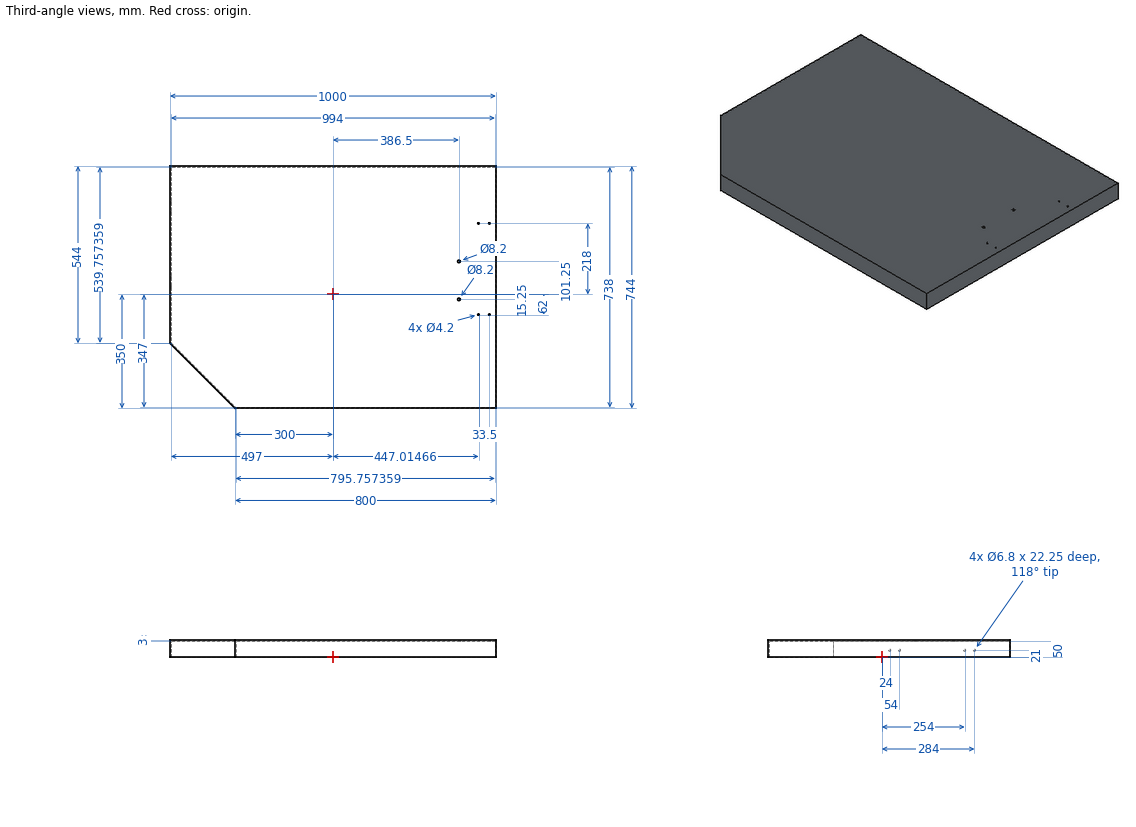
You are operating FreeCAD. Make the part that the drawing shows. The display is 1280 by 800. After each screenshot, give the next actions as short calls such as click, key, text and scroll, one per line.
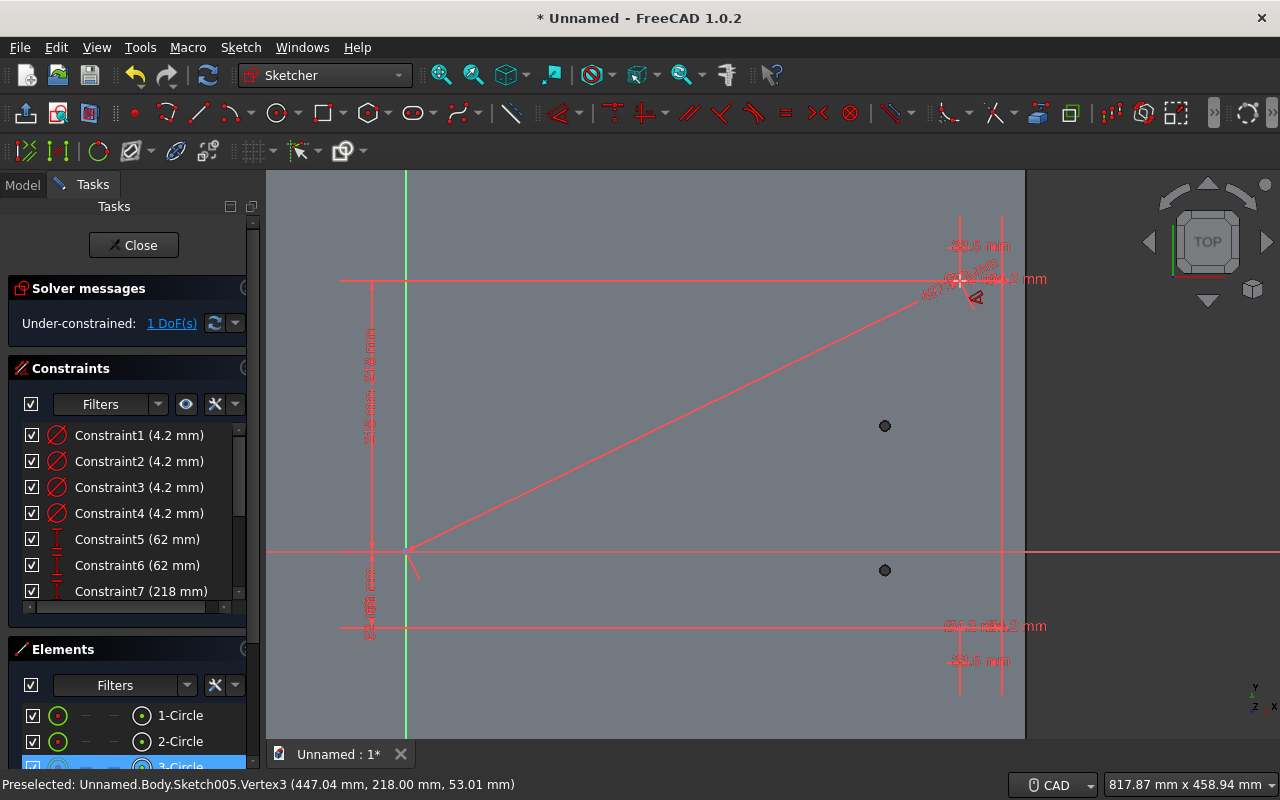
click(1002, 281)
click(981, 315)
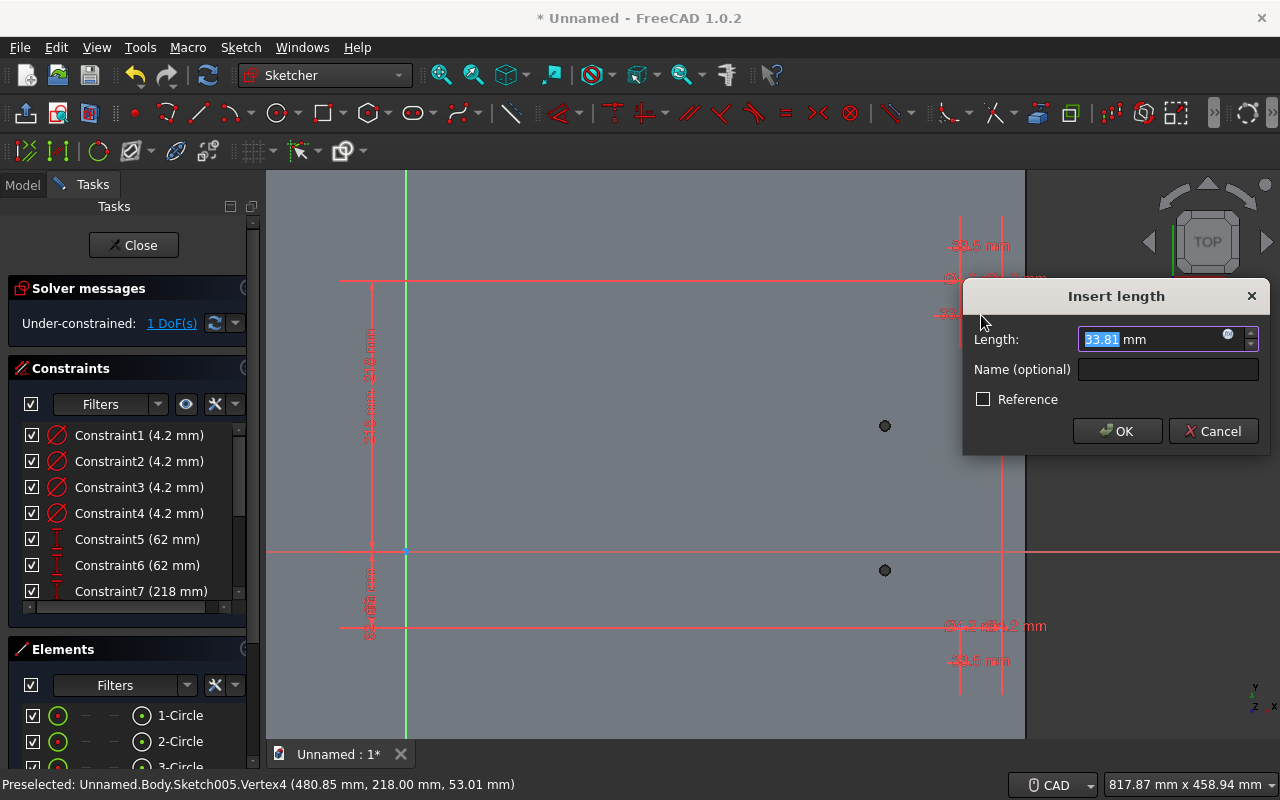
text(33.5)
key(Return)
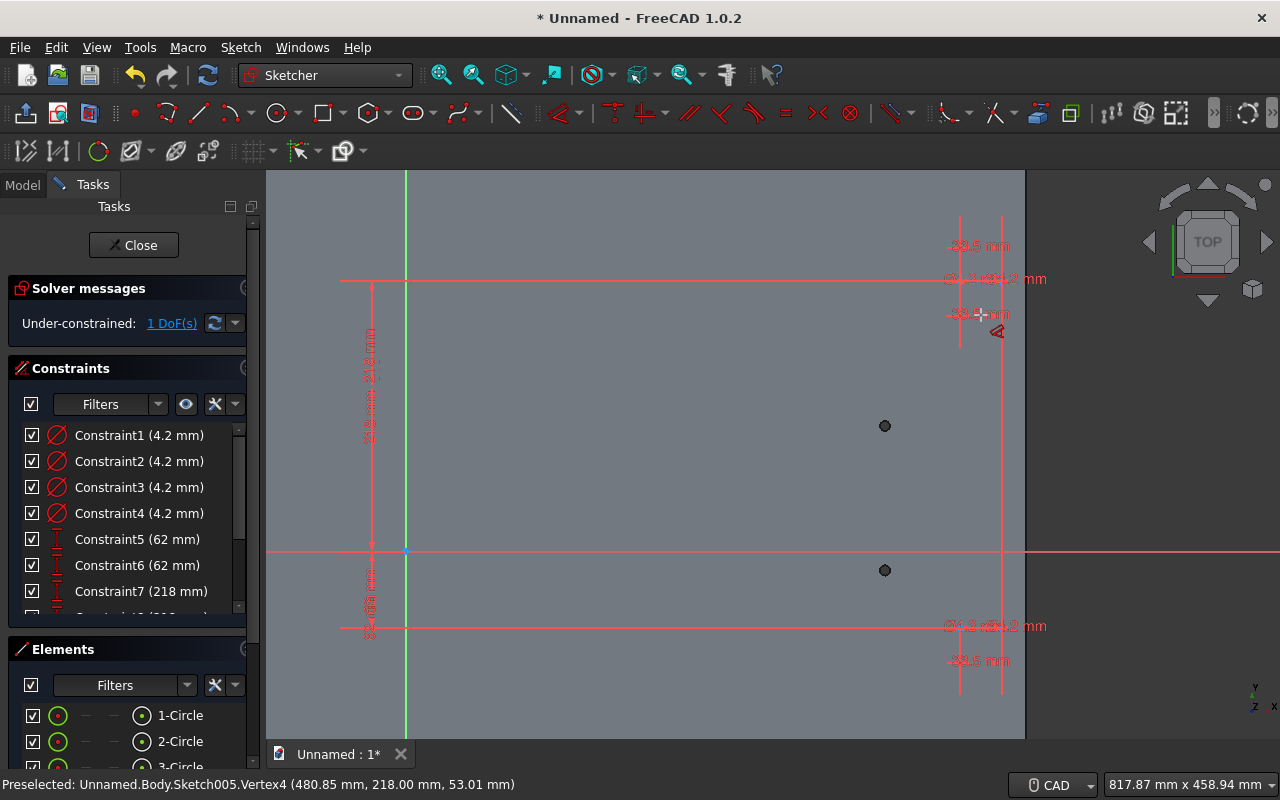
click(960, 628)
click(683, 662)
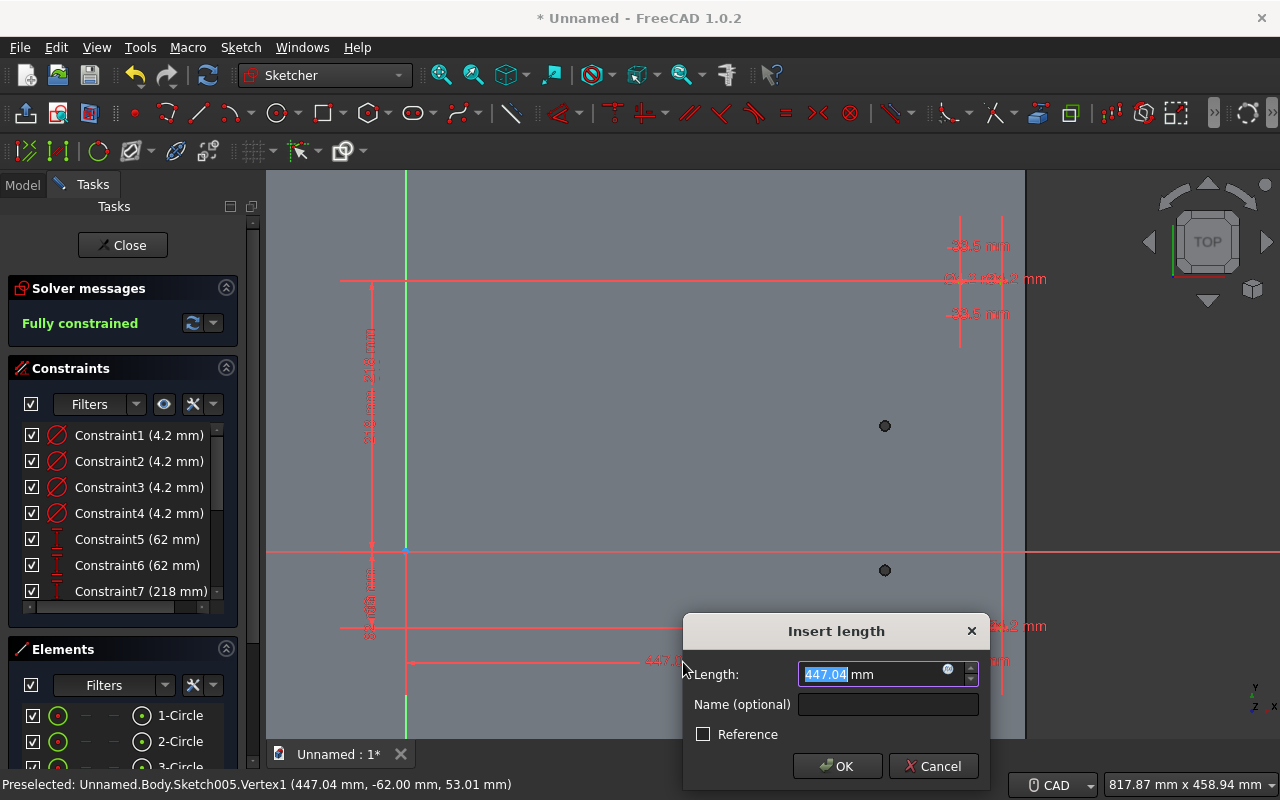
text(447.01466)
key(Return)
key(Escape)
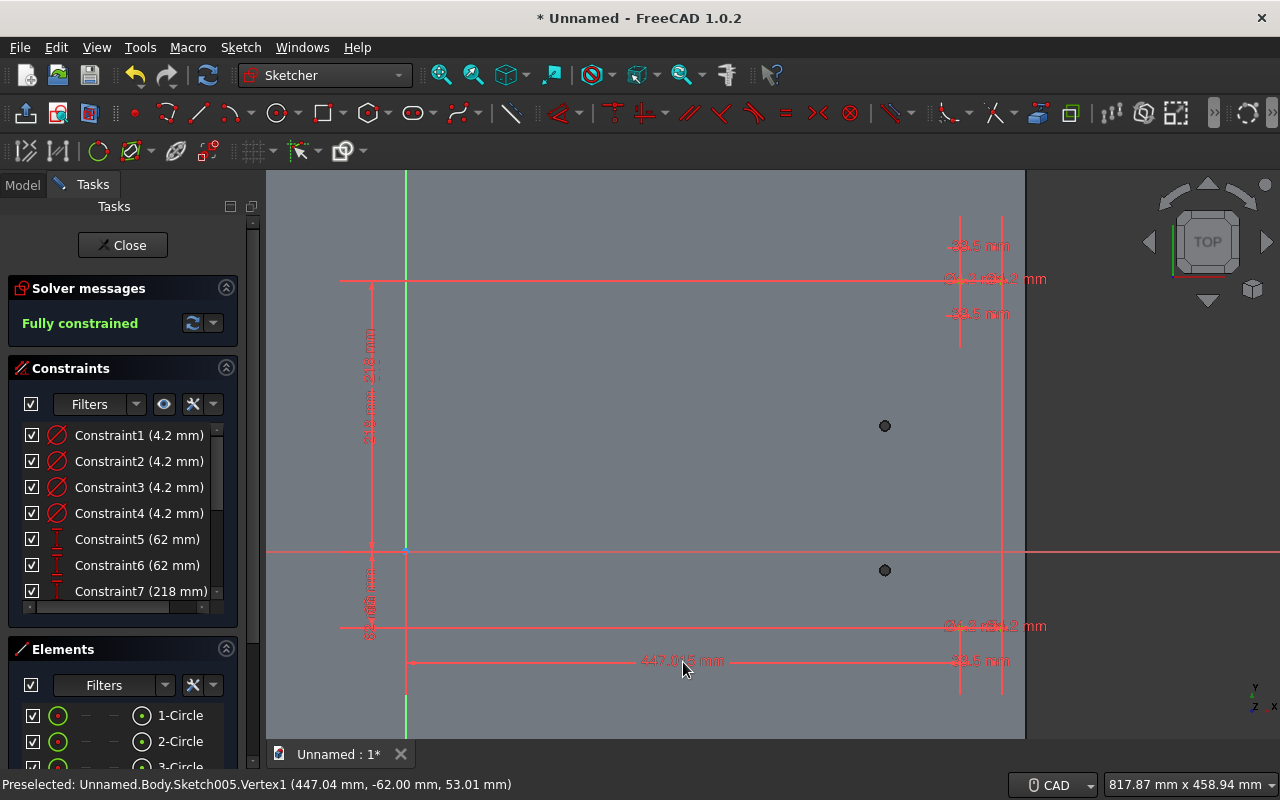
click(123, 245)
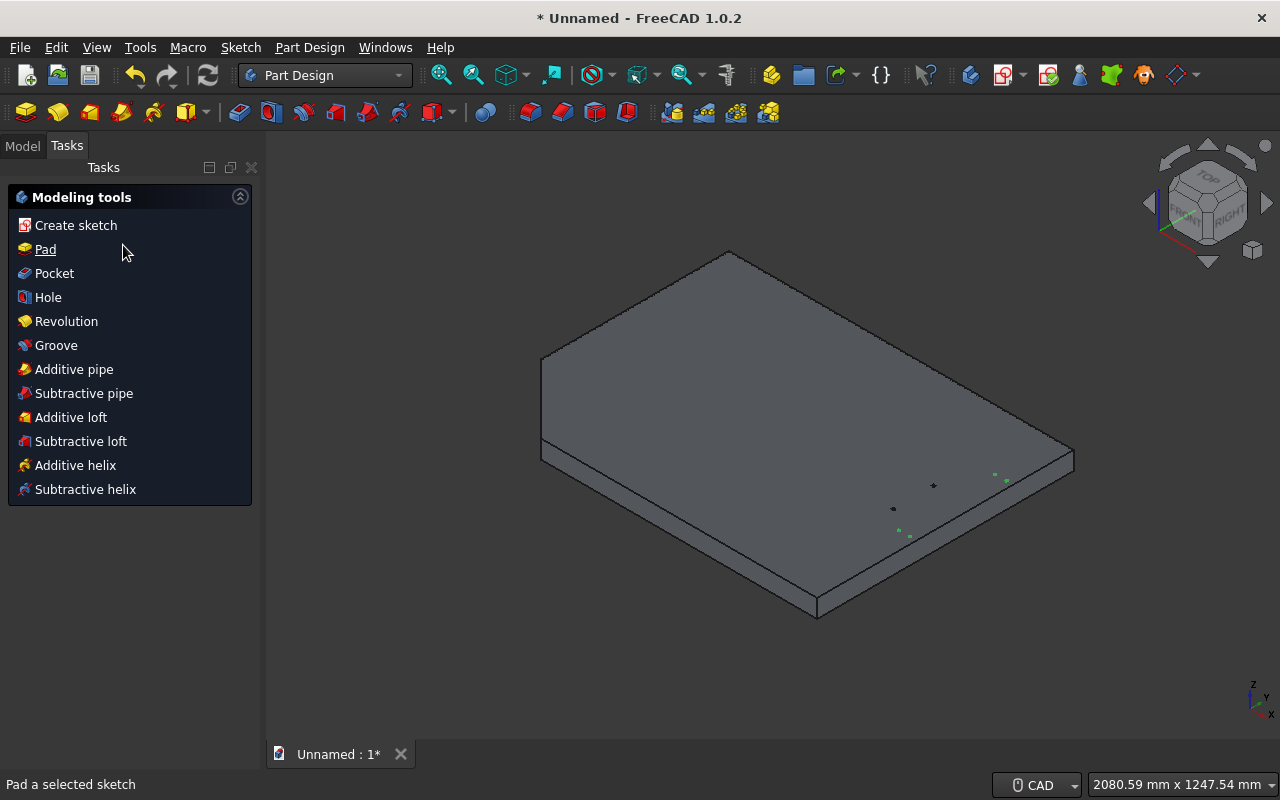
click(240, 112)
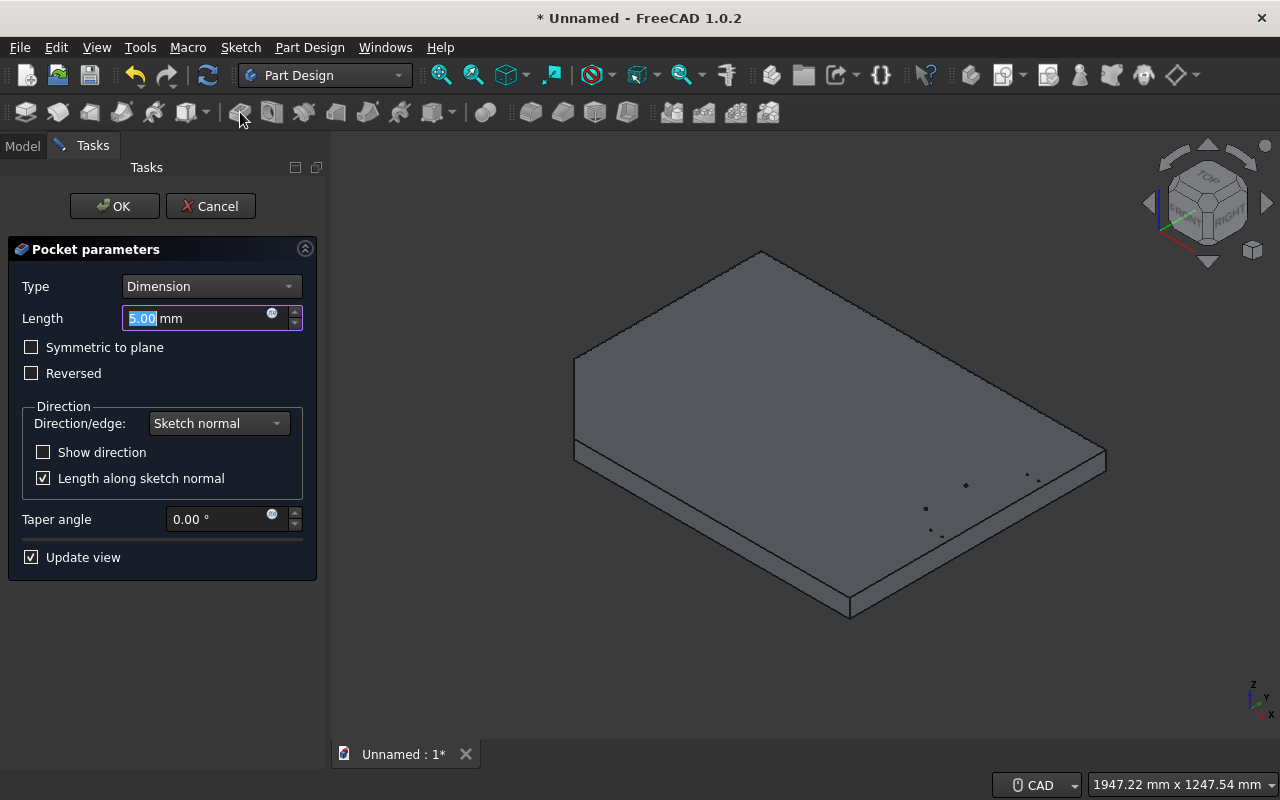
click(212, 286)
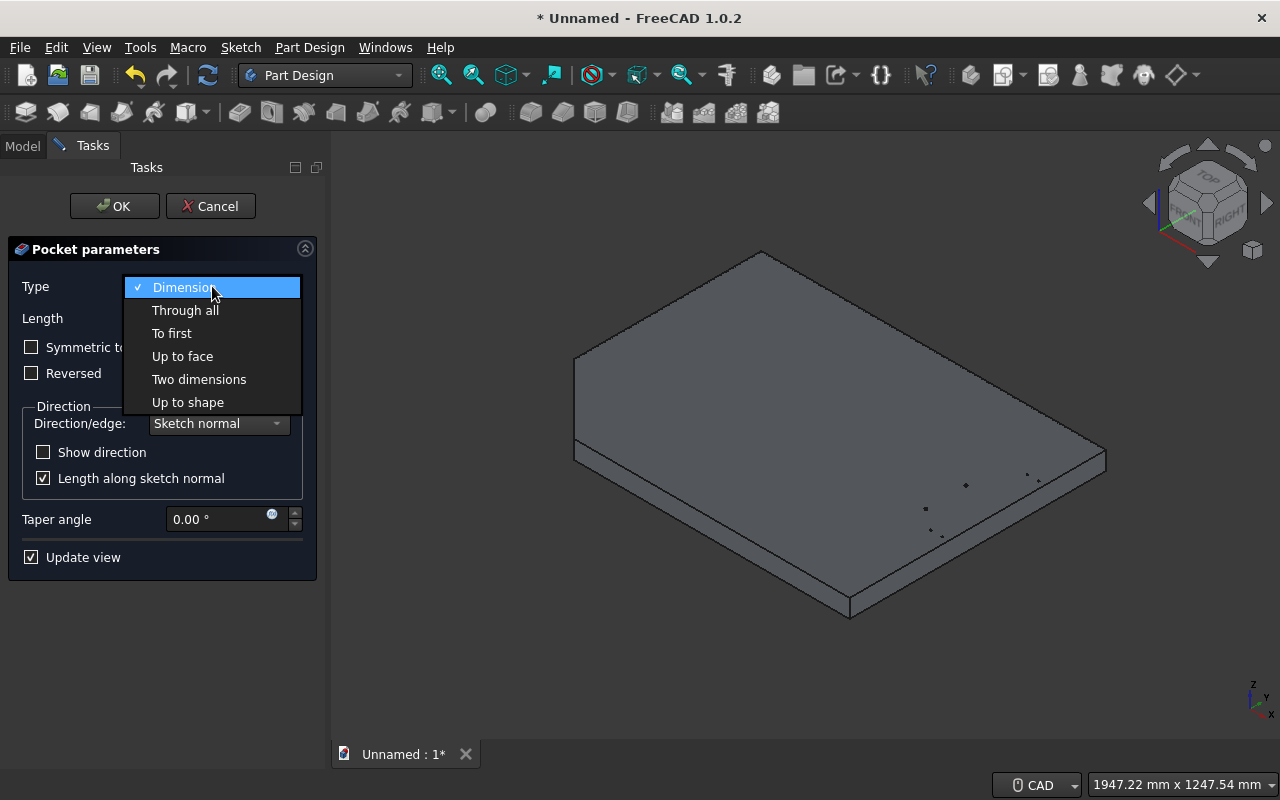
click(212, 310)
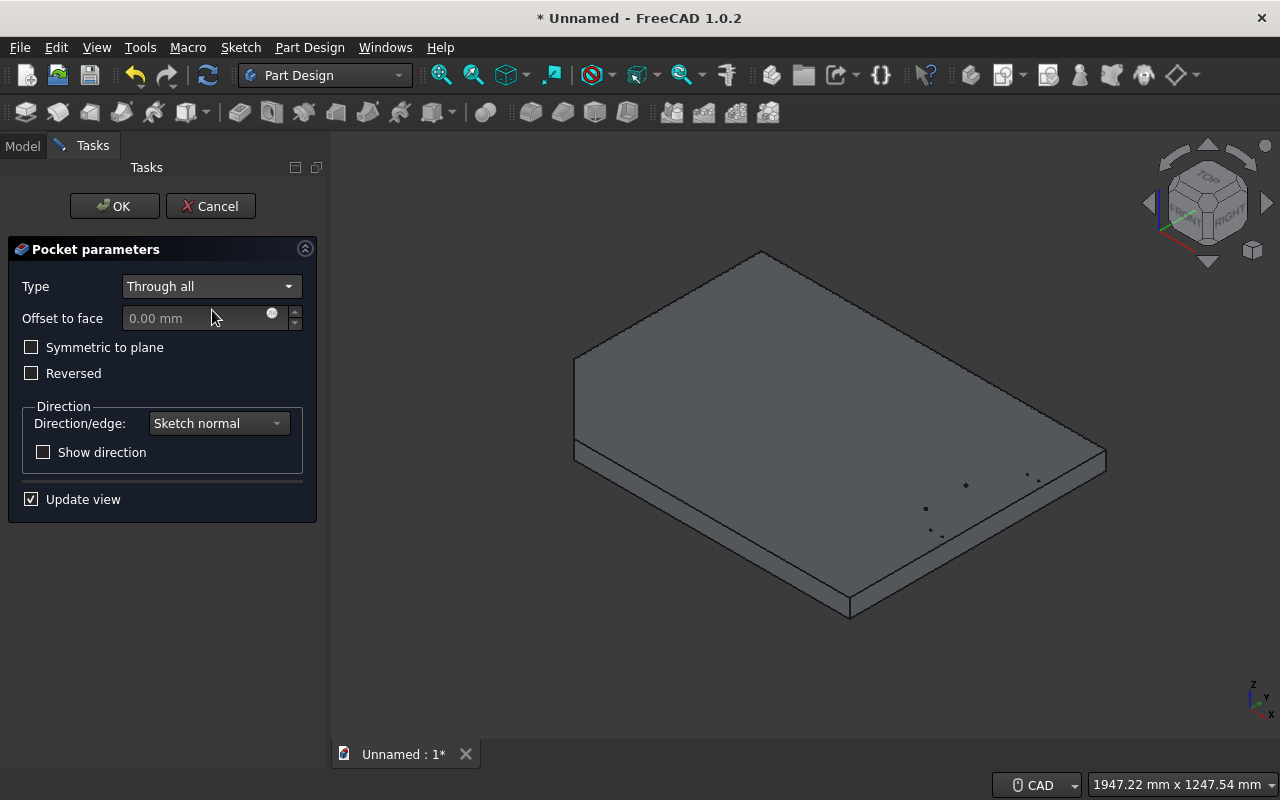
click(115, 206)